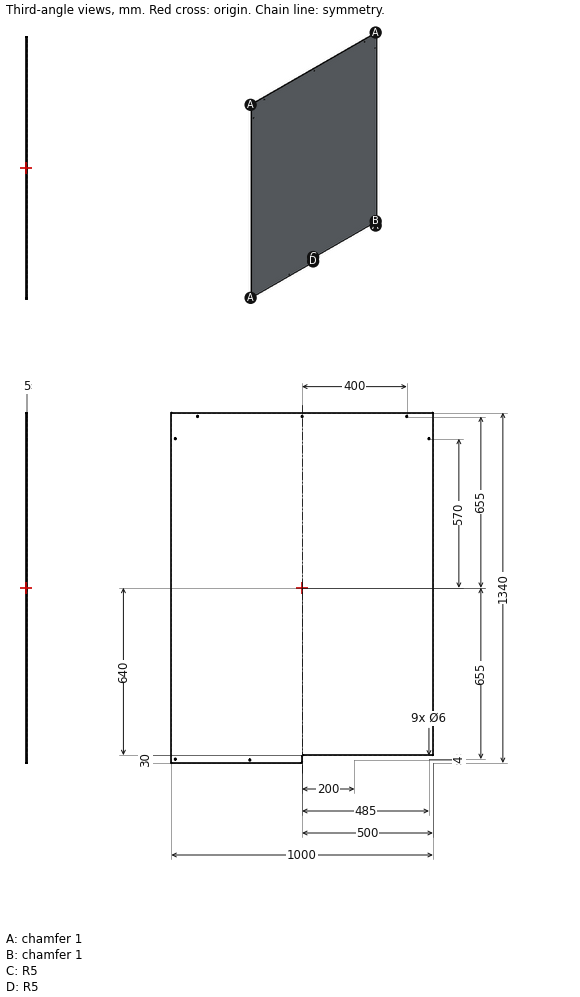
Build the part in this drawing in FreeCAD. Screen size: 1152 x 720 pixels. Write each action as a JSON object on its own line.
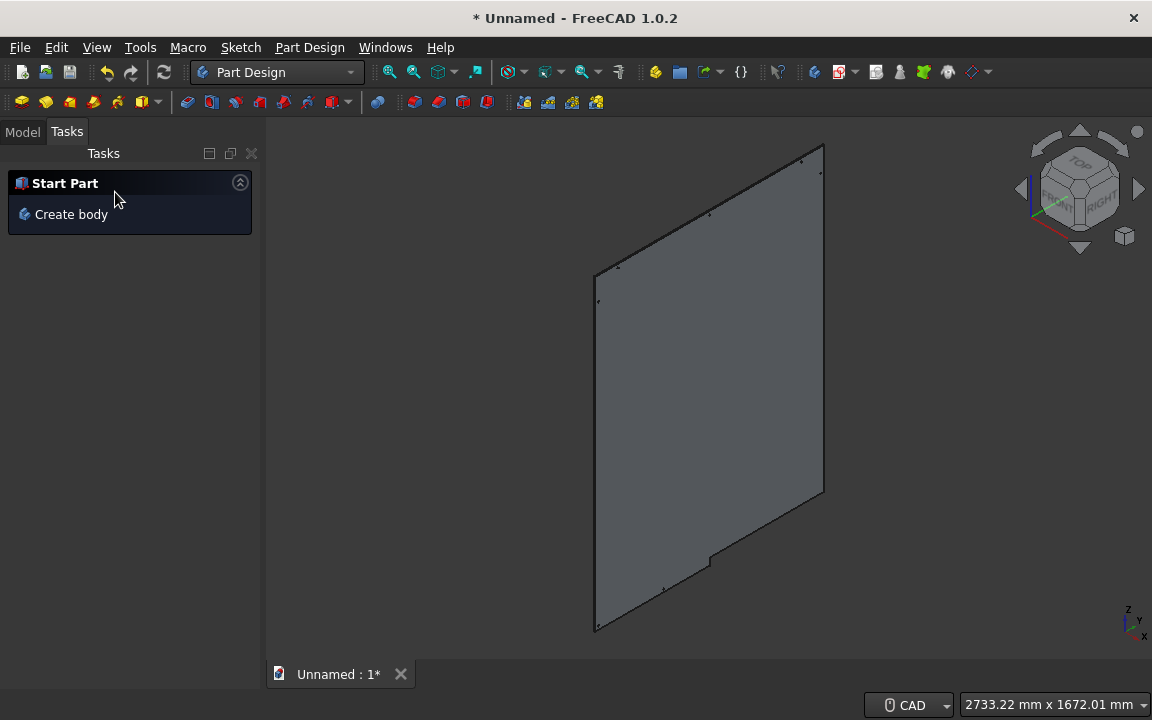
{"action": "scroll", "coordinate": [824, 490], "scroll_direction": "up", "scroll_amount": 15}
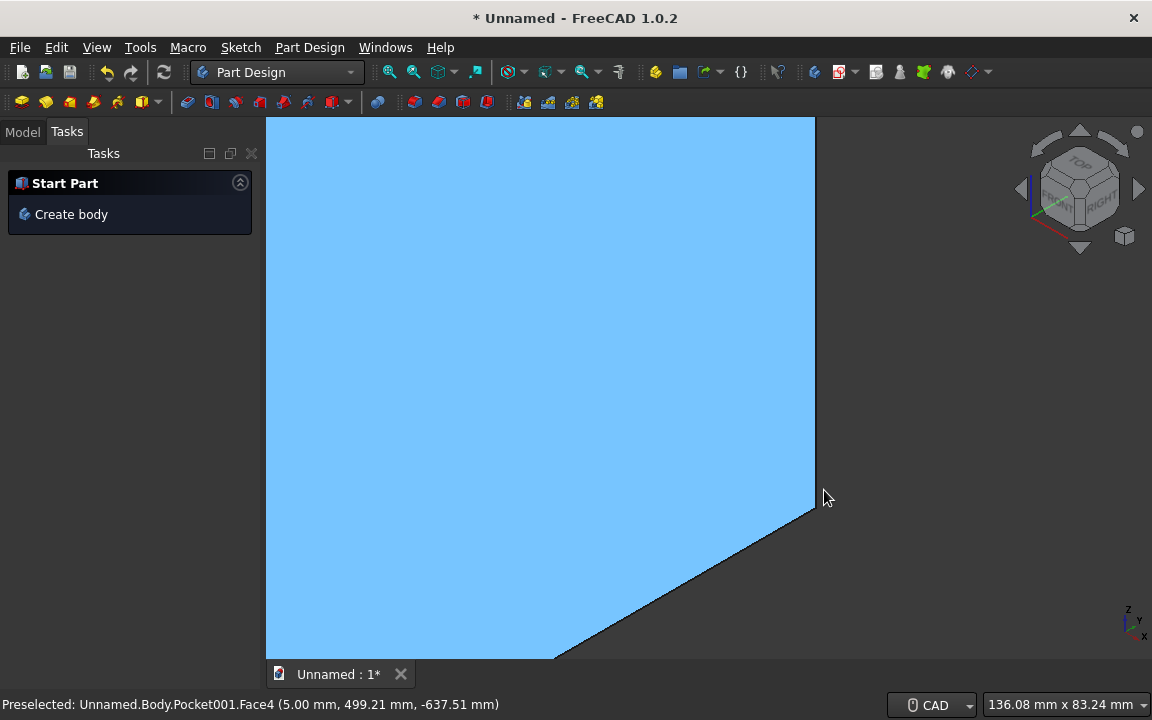
{"action": "left_click", "coordinate": [390, 72]}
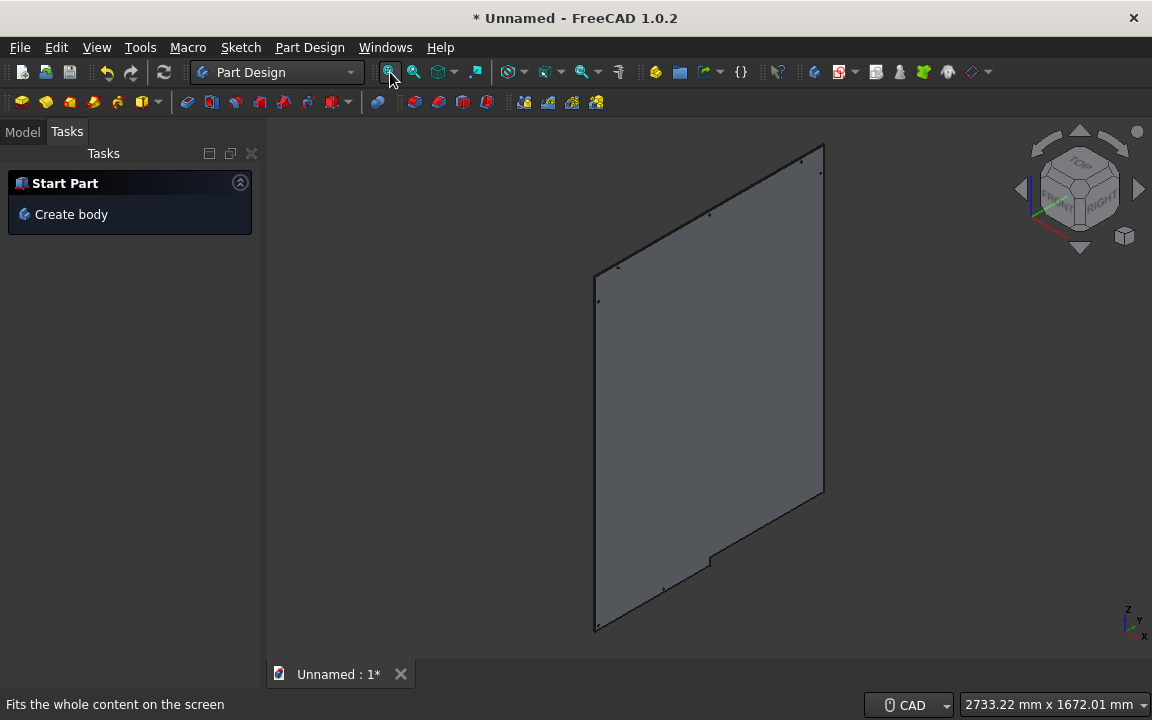
{"action": "key", "text": "2"}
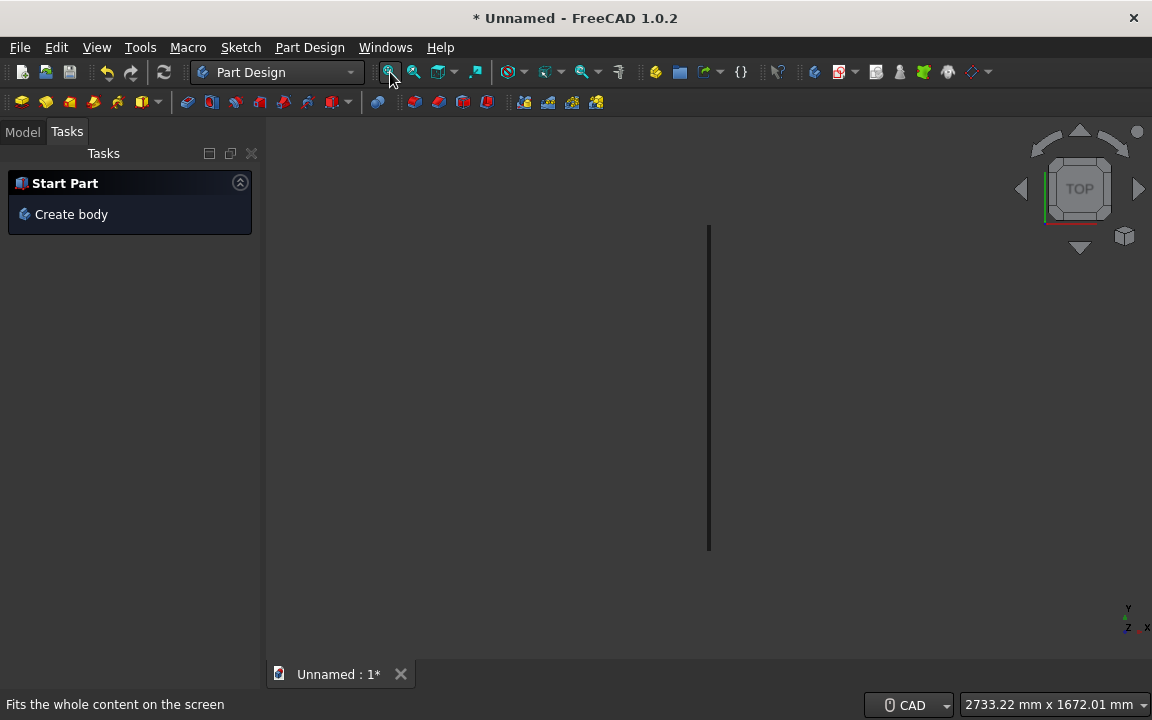
{"action": "scroll", "coordinate": [709, 225], "scroll_direction": "up", "scroll_amount": 15}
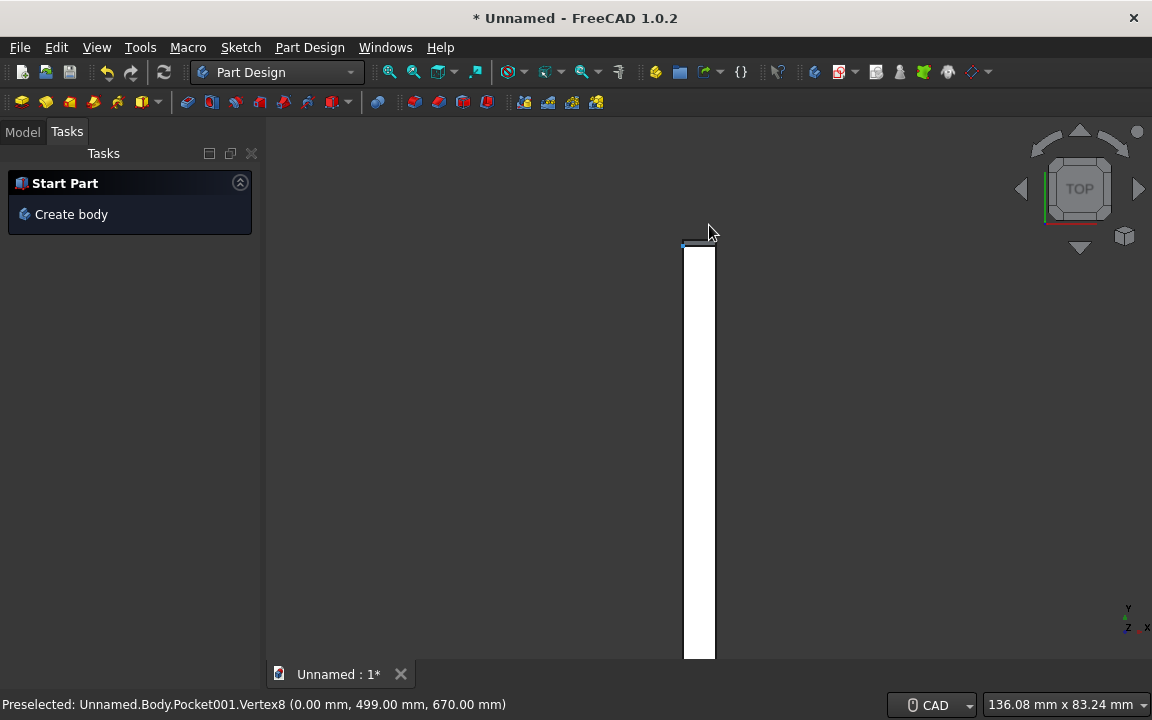
{"action": "left_click", "coordinate": [390, 72]}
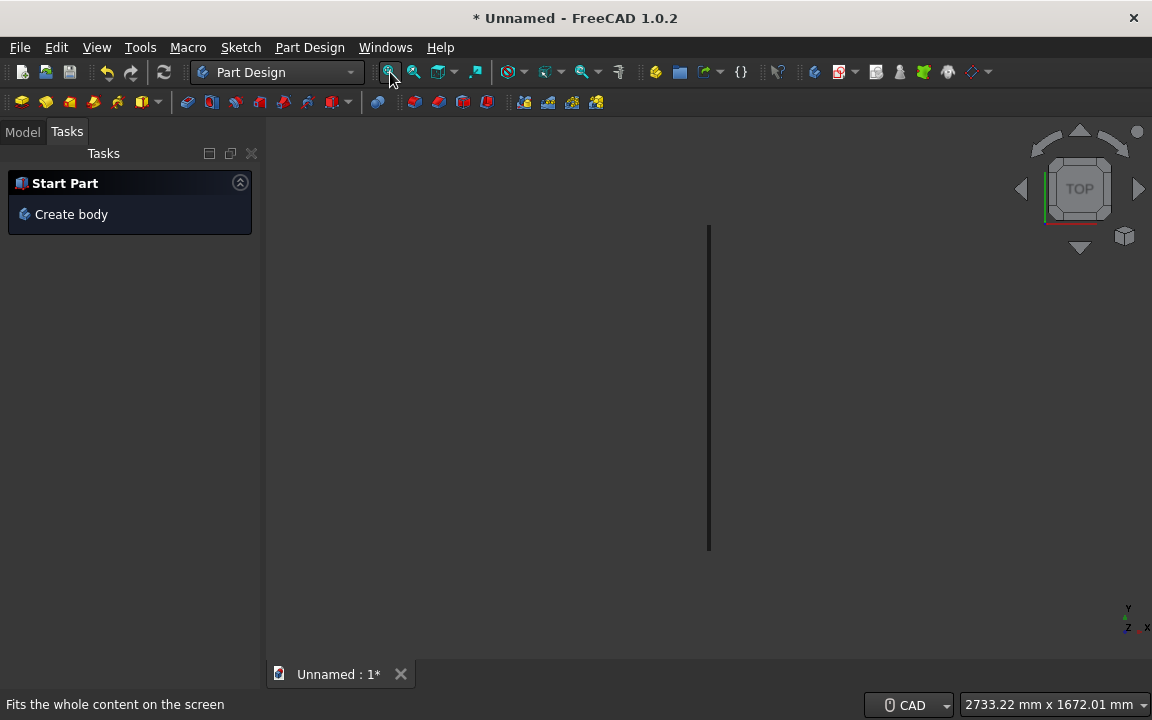
{"action": "key", "text": "0"}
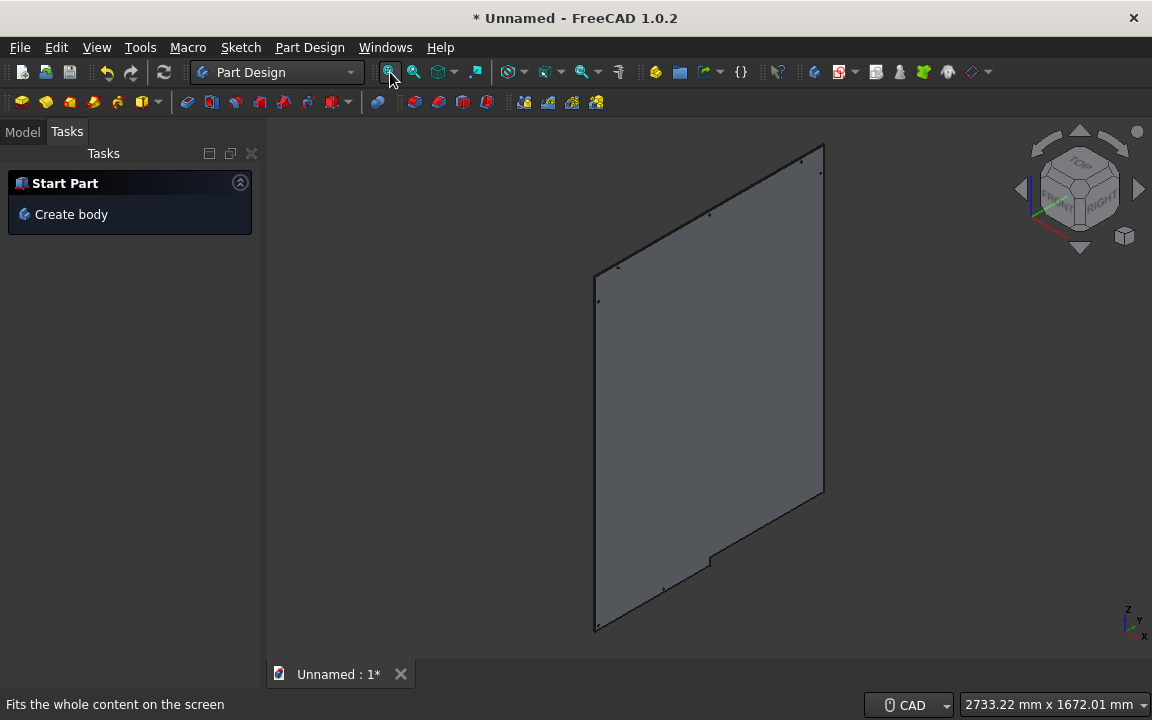
{"action": "scroll", "coordinate": [824, 490], "scroll_direction": "up", "scroll_amount": 15}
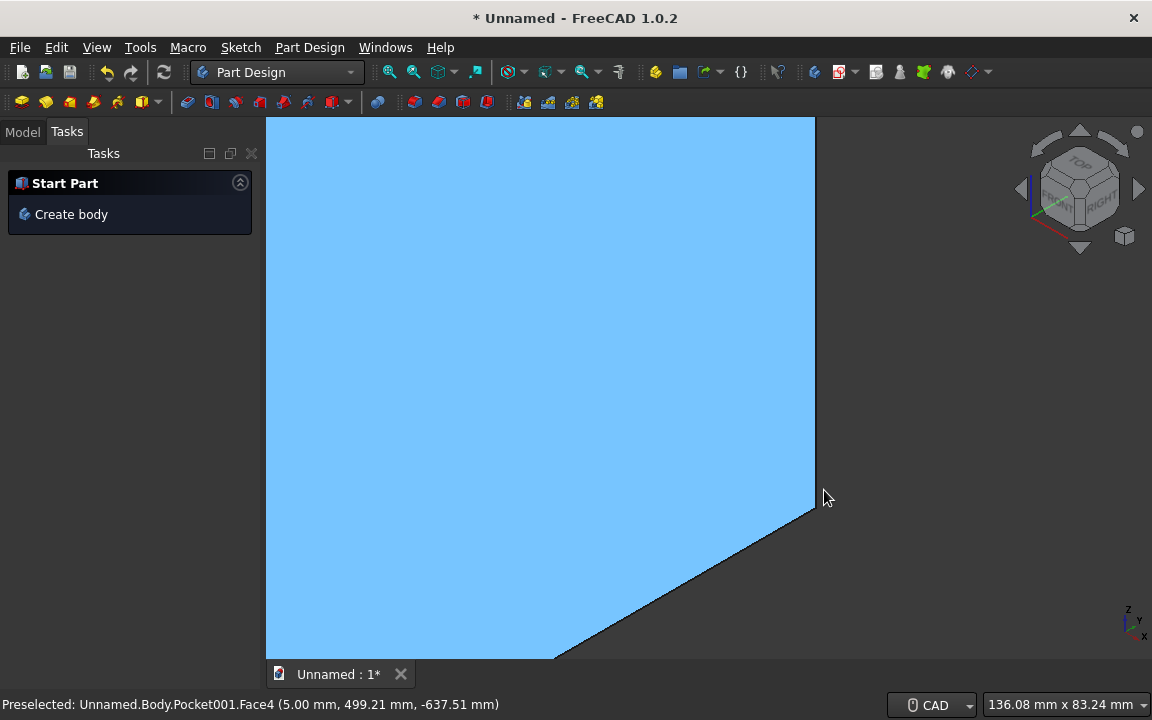
{"action": "left_click", "coordinate": [390, 72]}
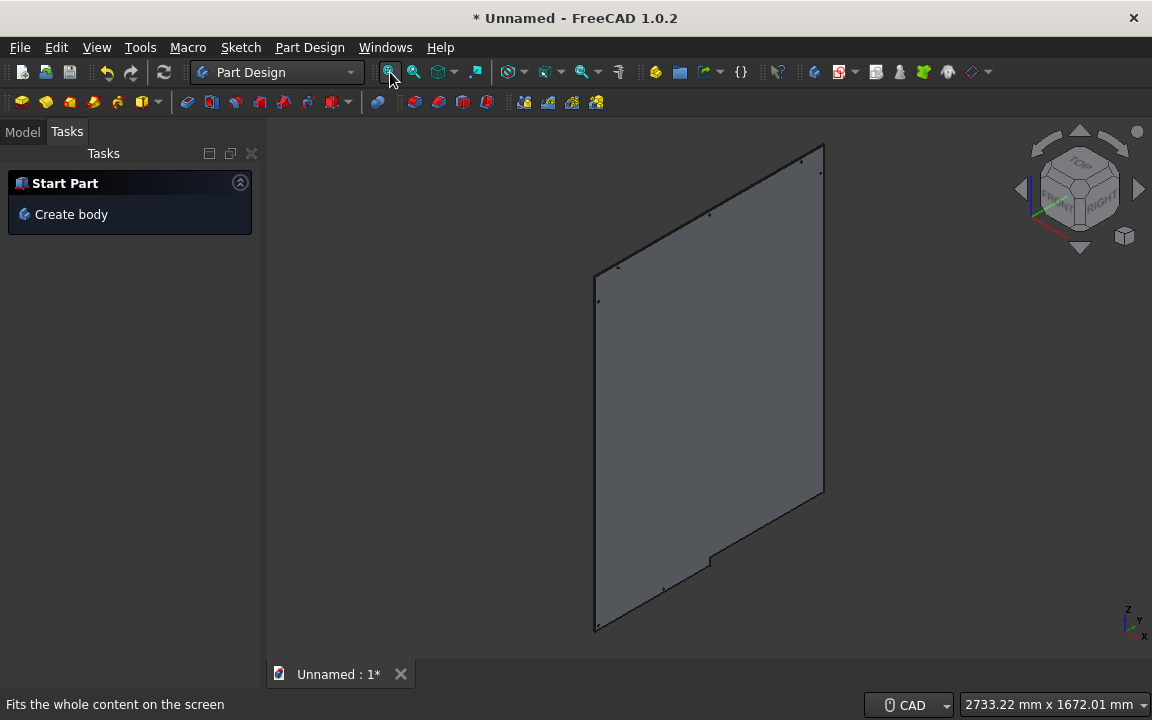
{"action": "key", "text": "1"}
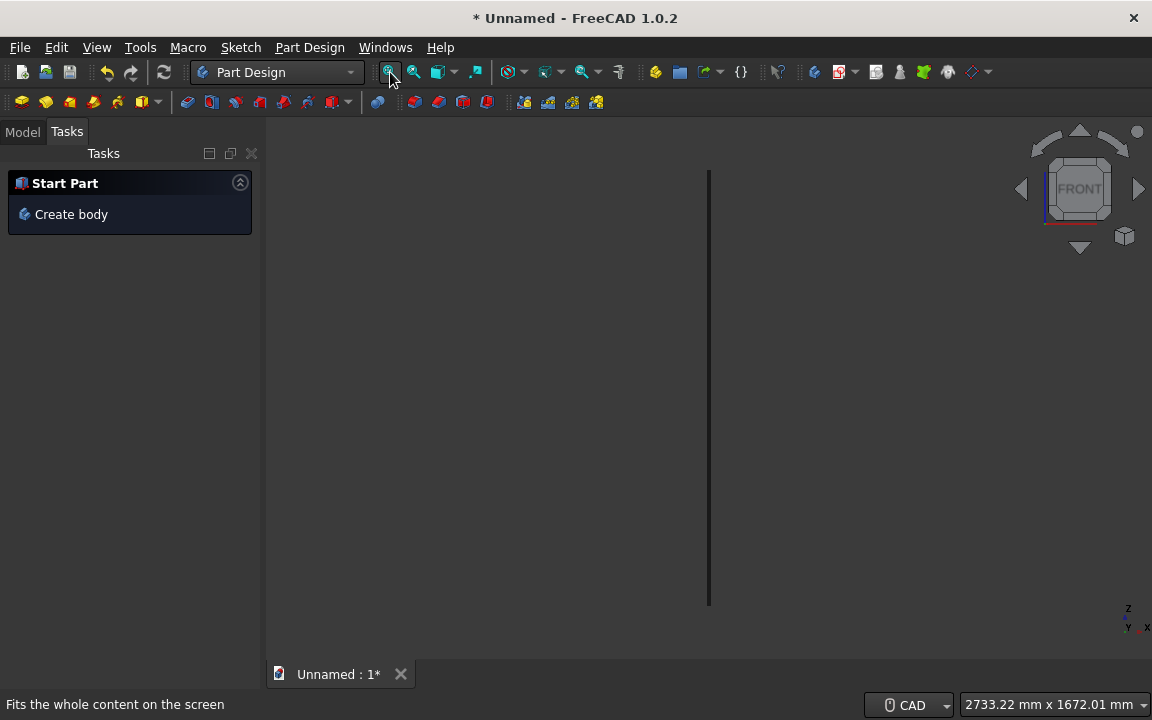
{"action": "scroll", "coordinate": [709, 594], "scroll_direction": "up", "scroll_amount": 15}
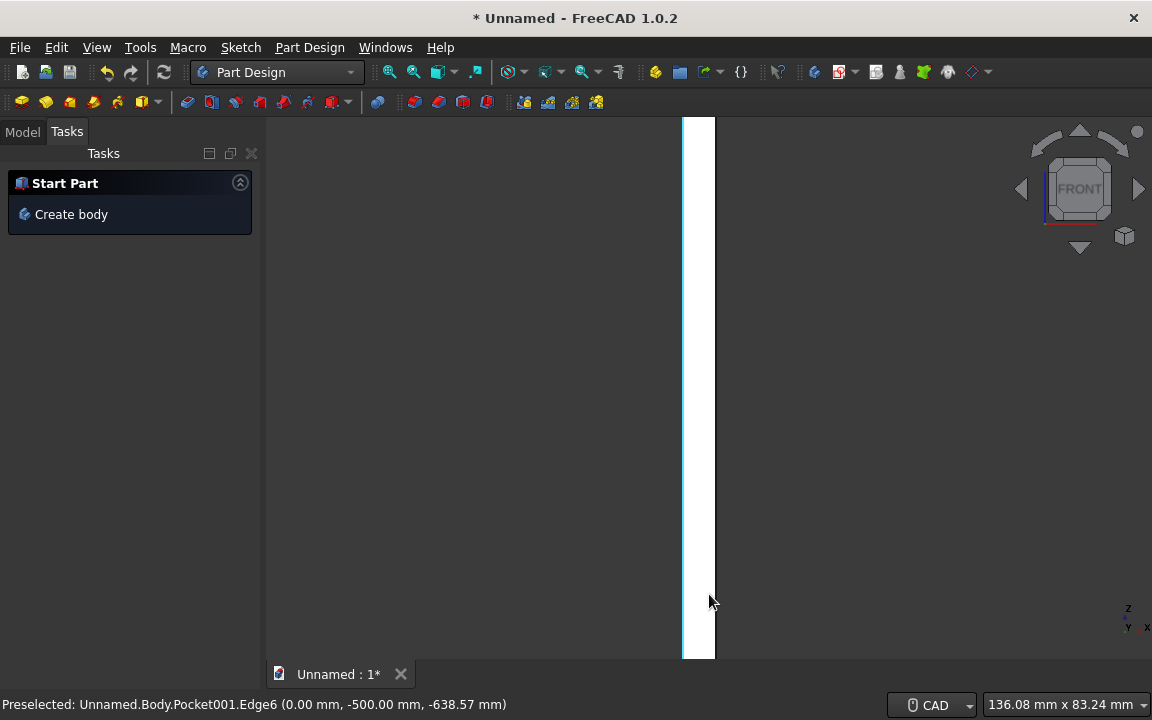
{"action": "left_click", "coordinate": [390, 72]}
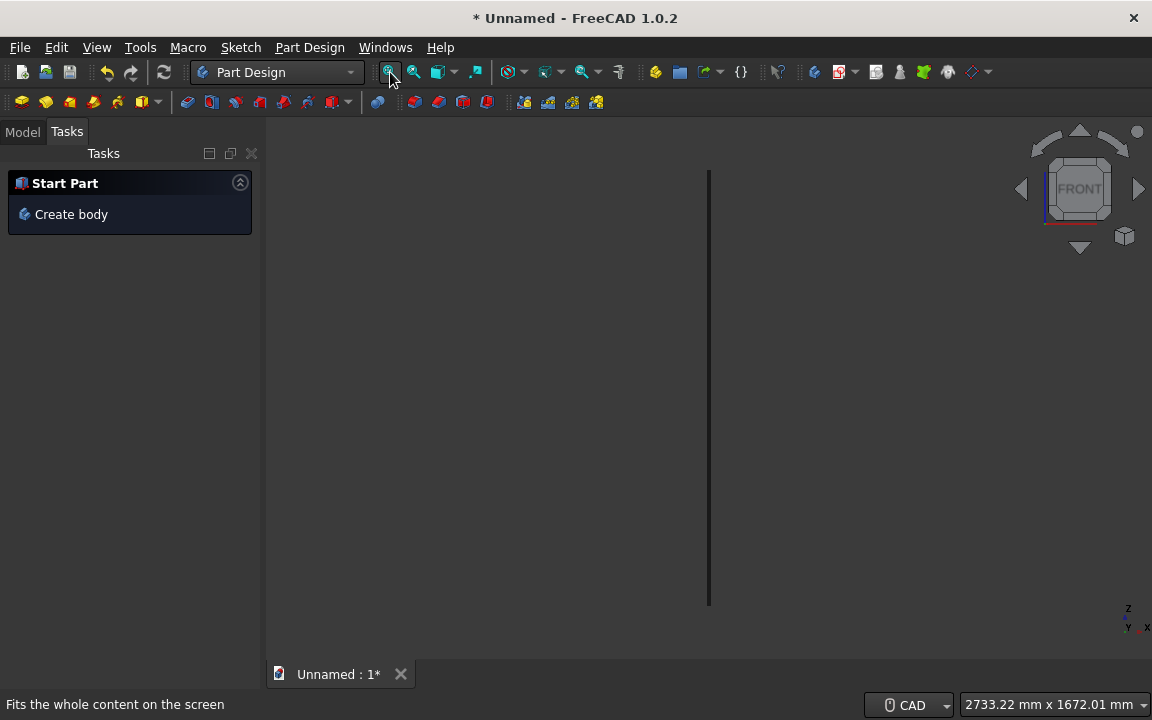
{"action": "key", "text": "3"}